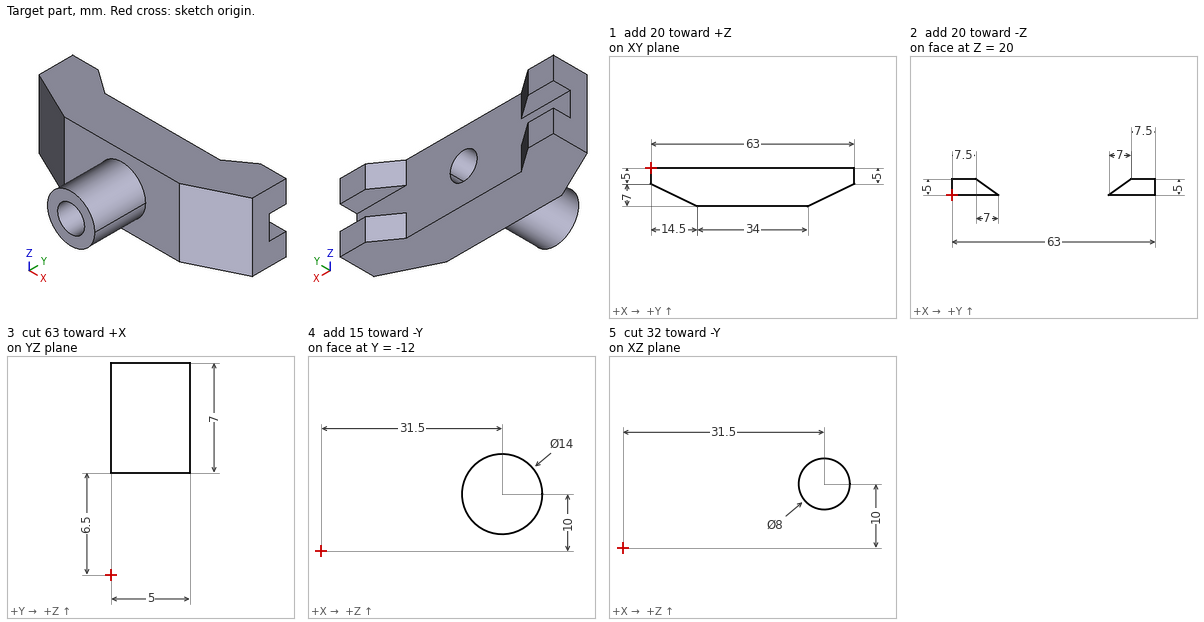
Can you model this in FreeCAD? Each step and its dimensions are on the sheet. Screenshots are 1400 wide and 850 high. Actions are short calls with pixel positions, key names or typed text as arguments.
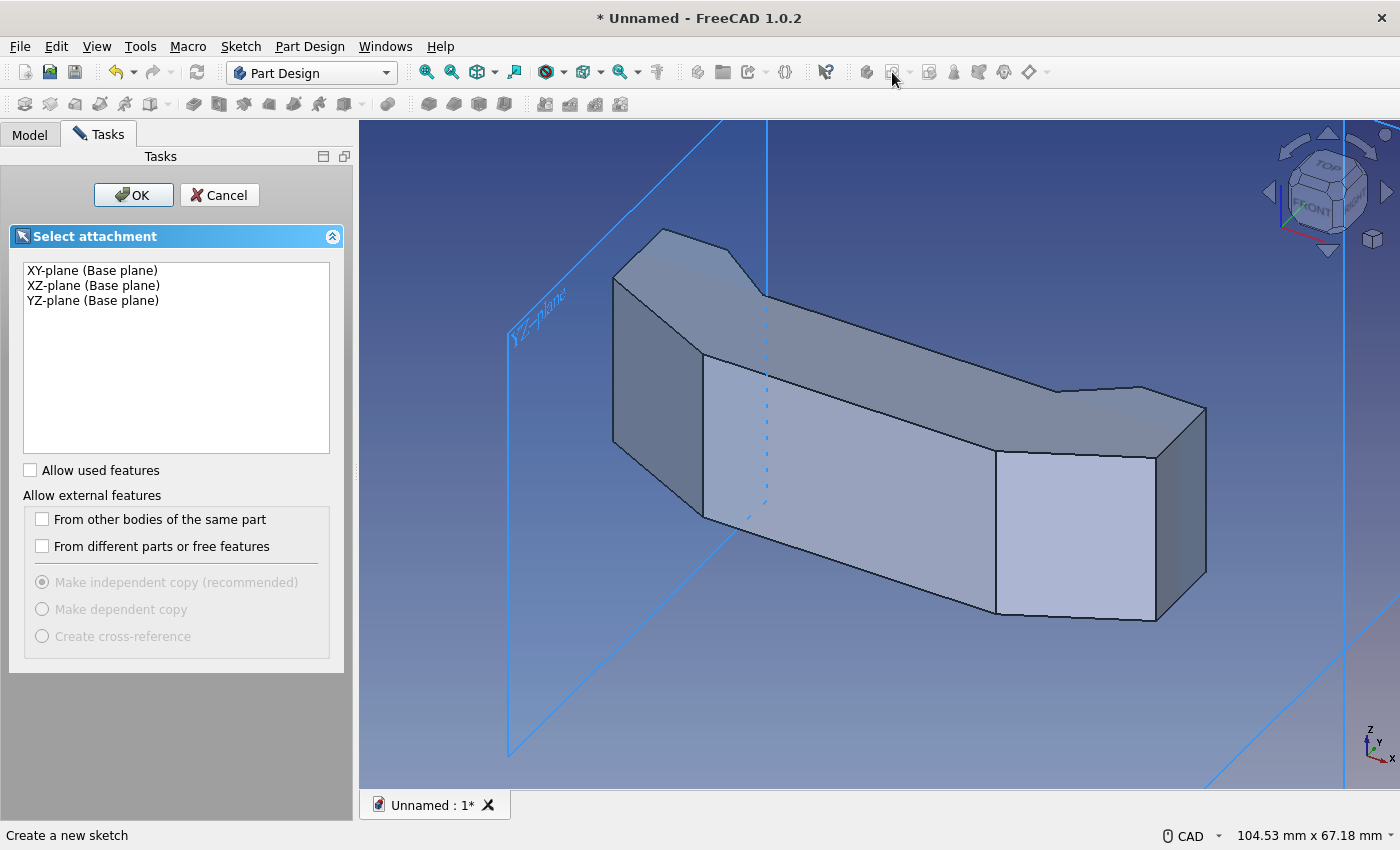
click(84, 300)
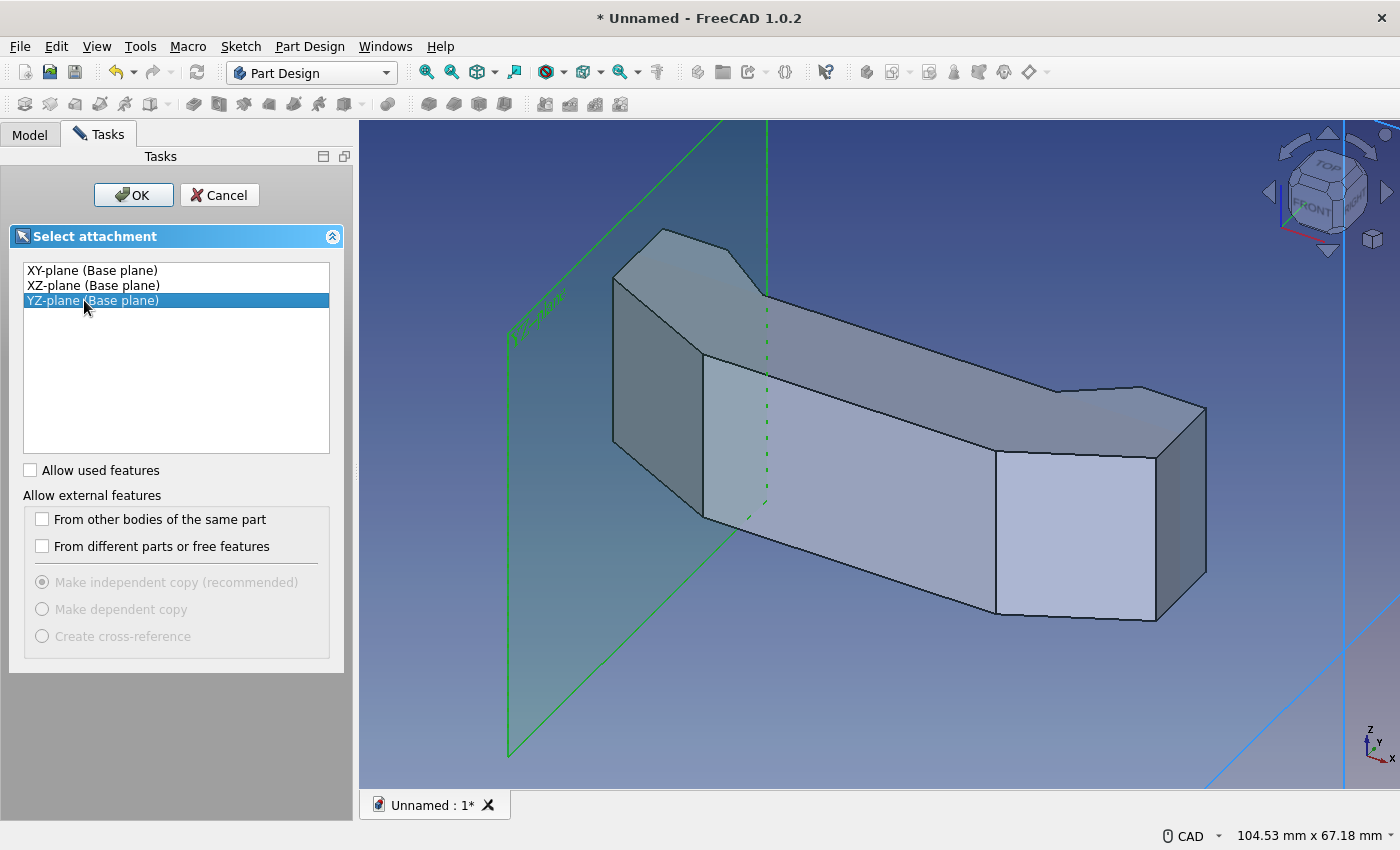
click(134, 195)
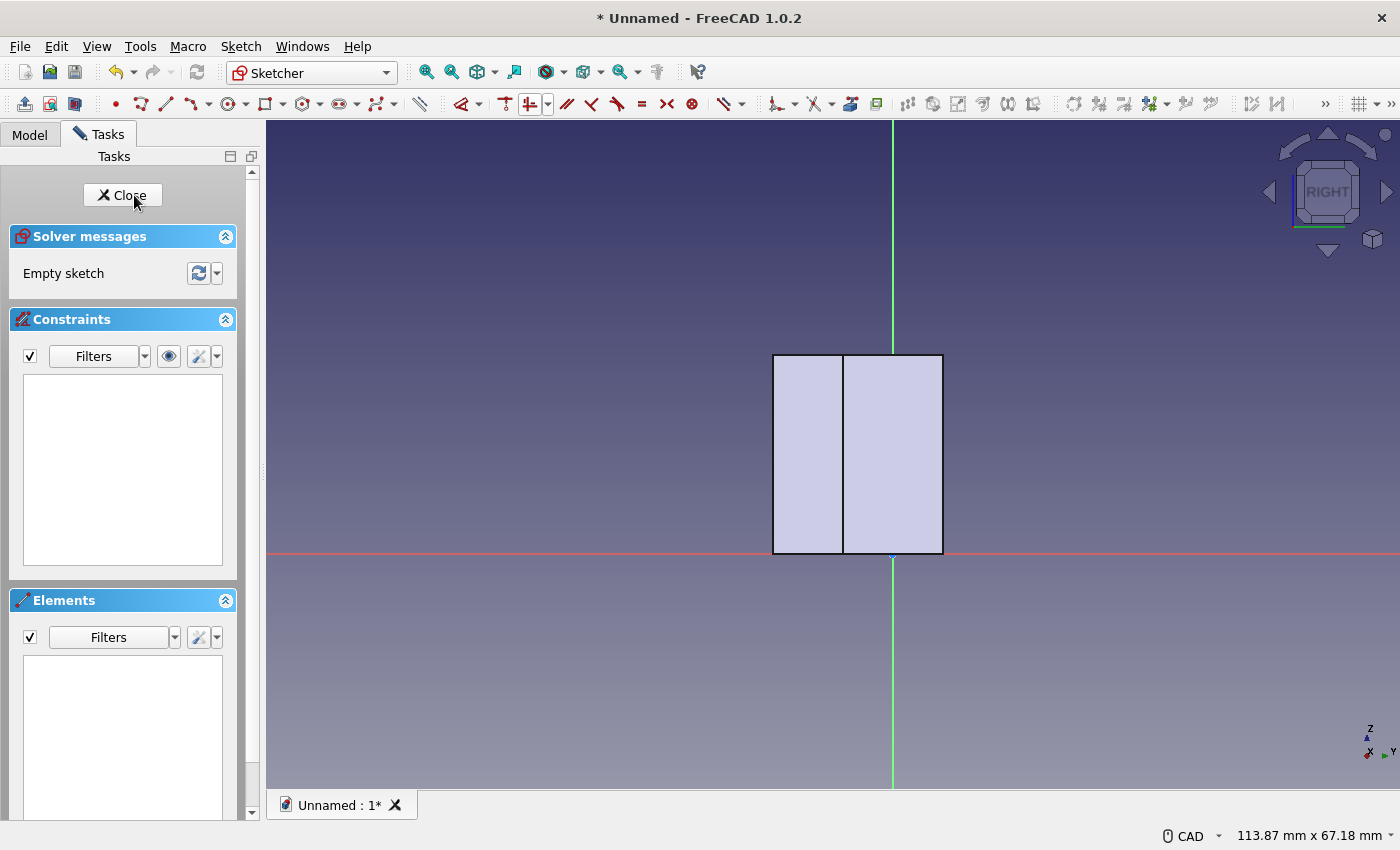
click(75, 104)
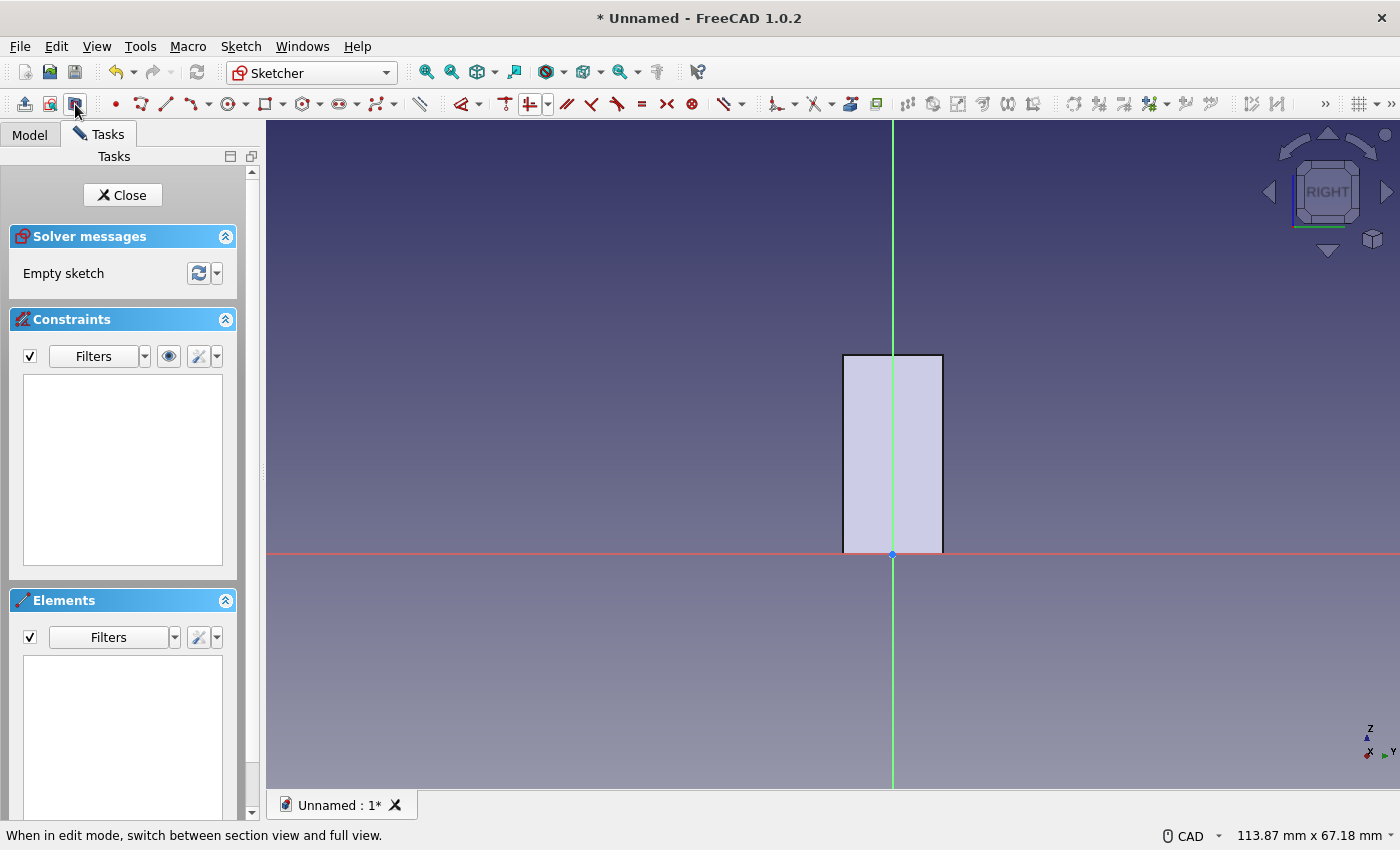
scroll(984, 501, up, 6)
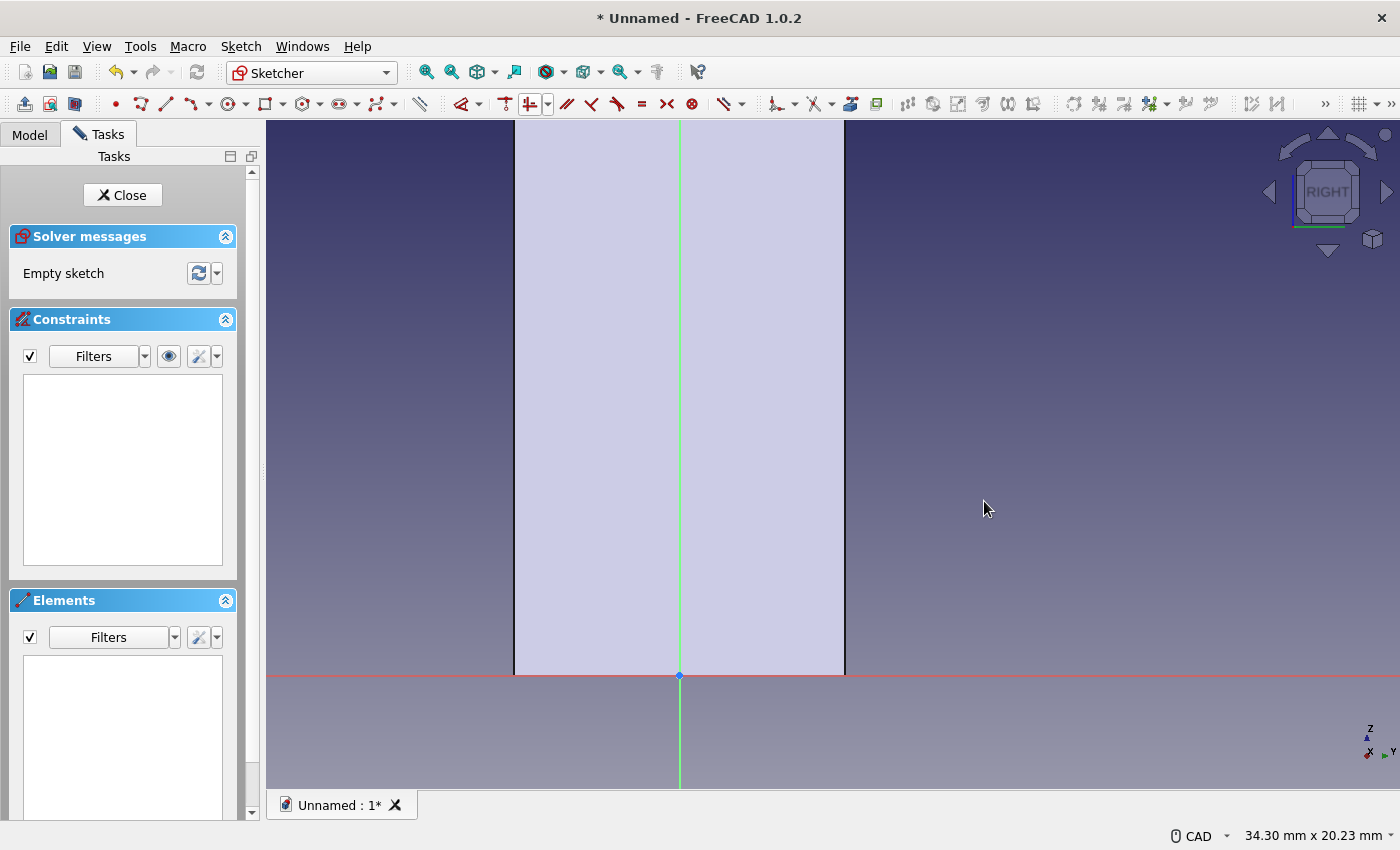
click(264, 104)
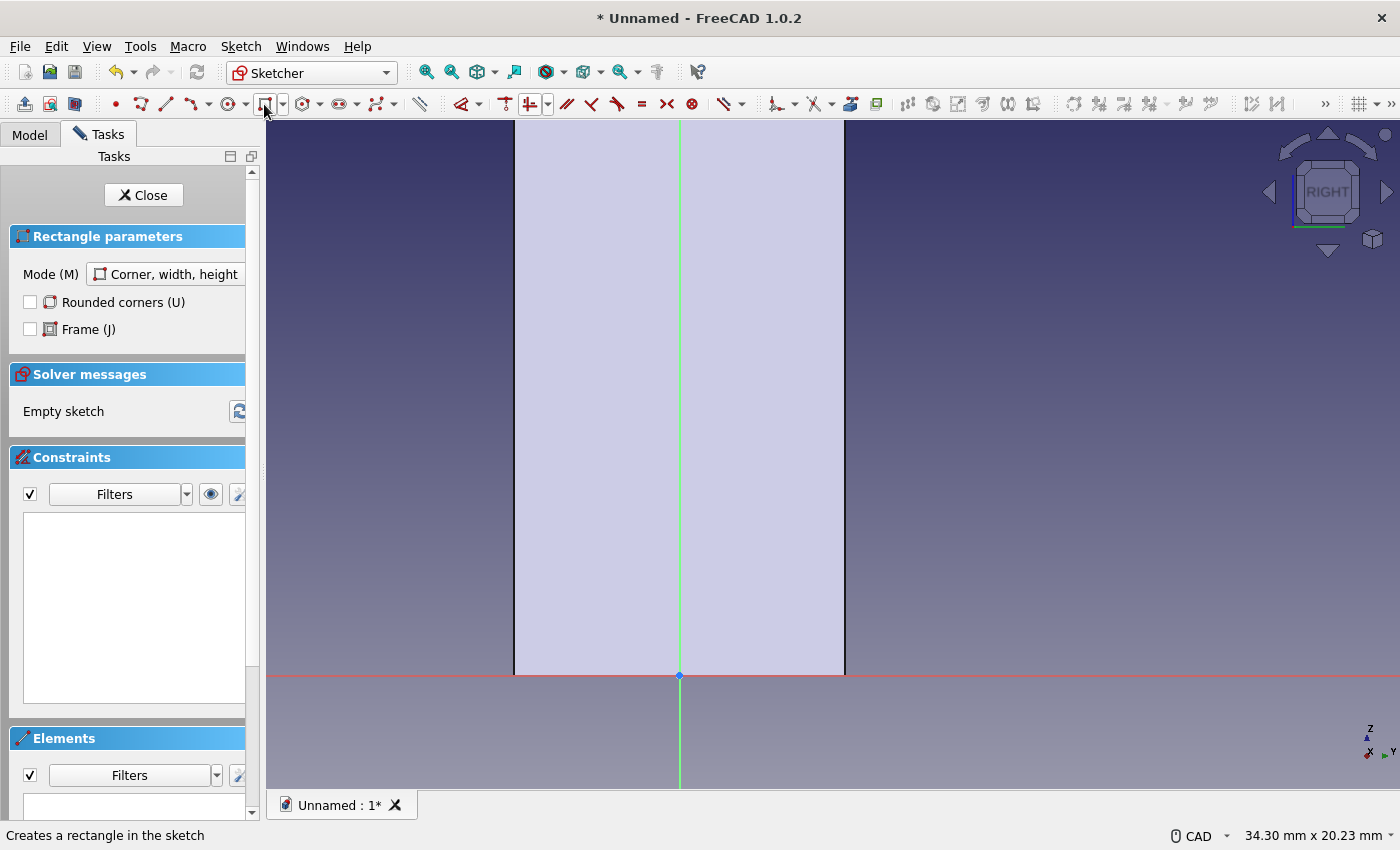
click(680, 230)
move(845, 461)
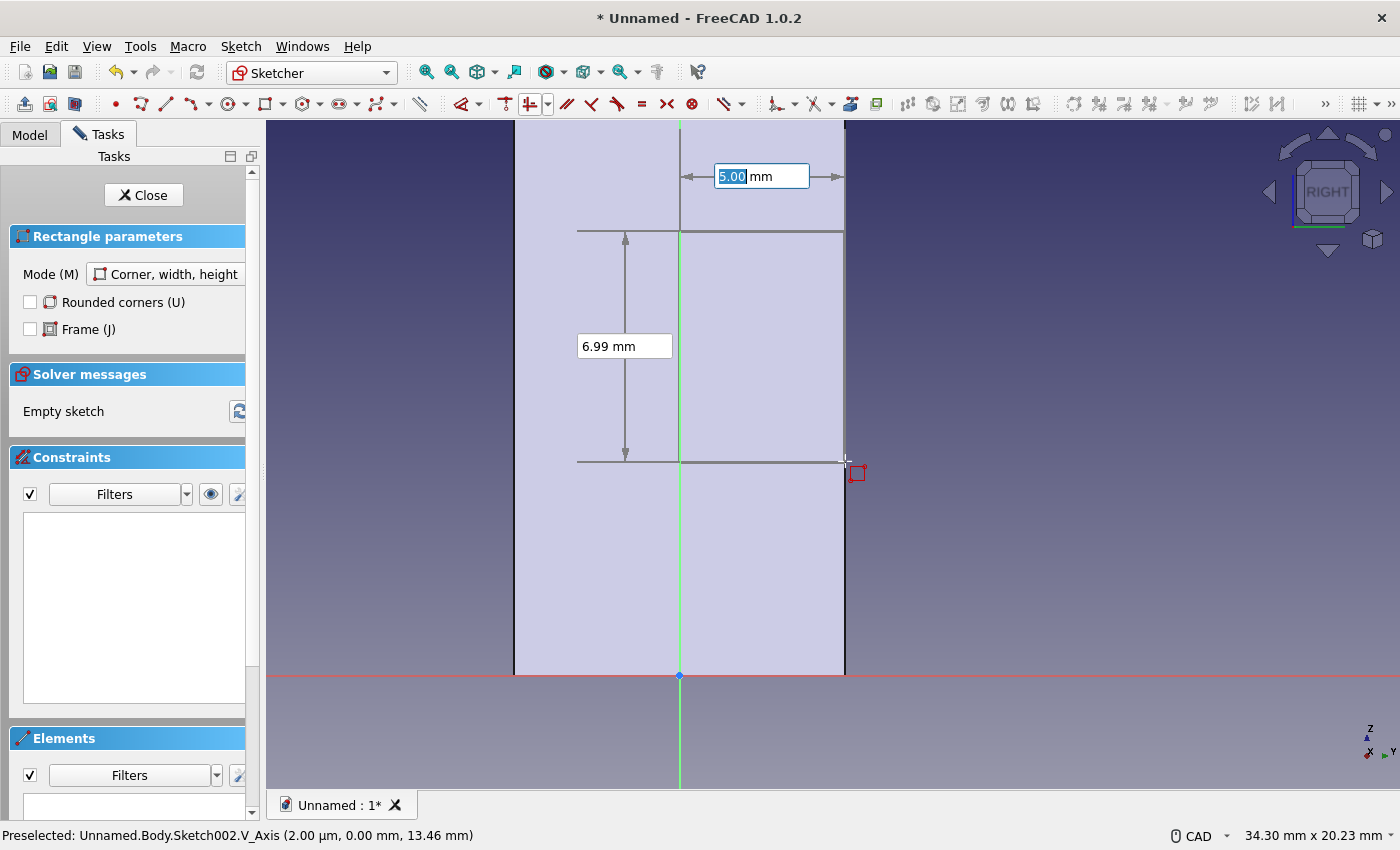
text(5)
key(Tab)
text(7)
key(Return)
key(Escape)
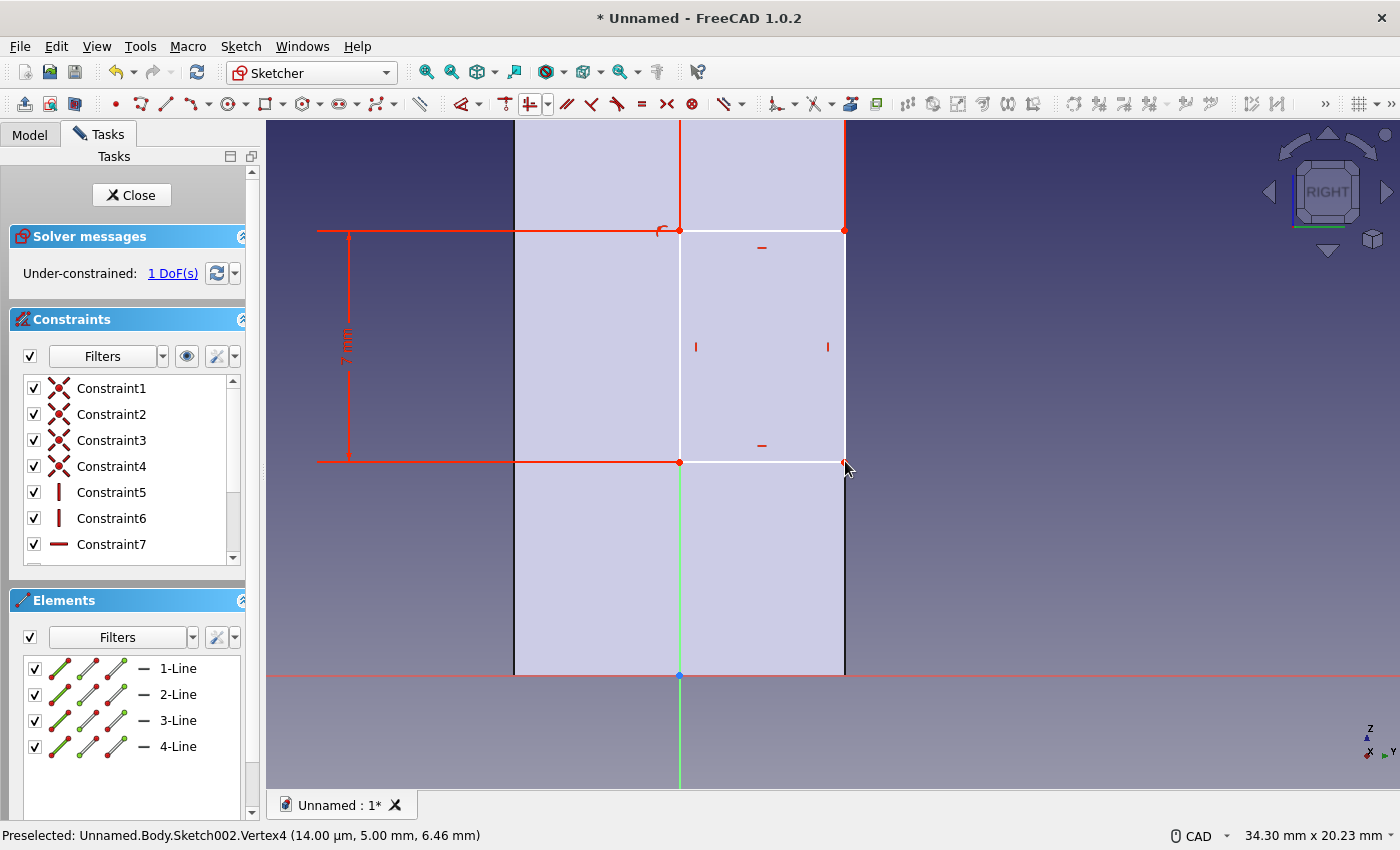
click(460, 104)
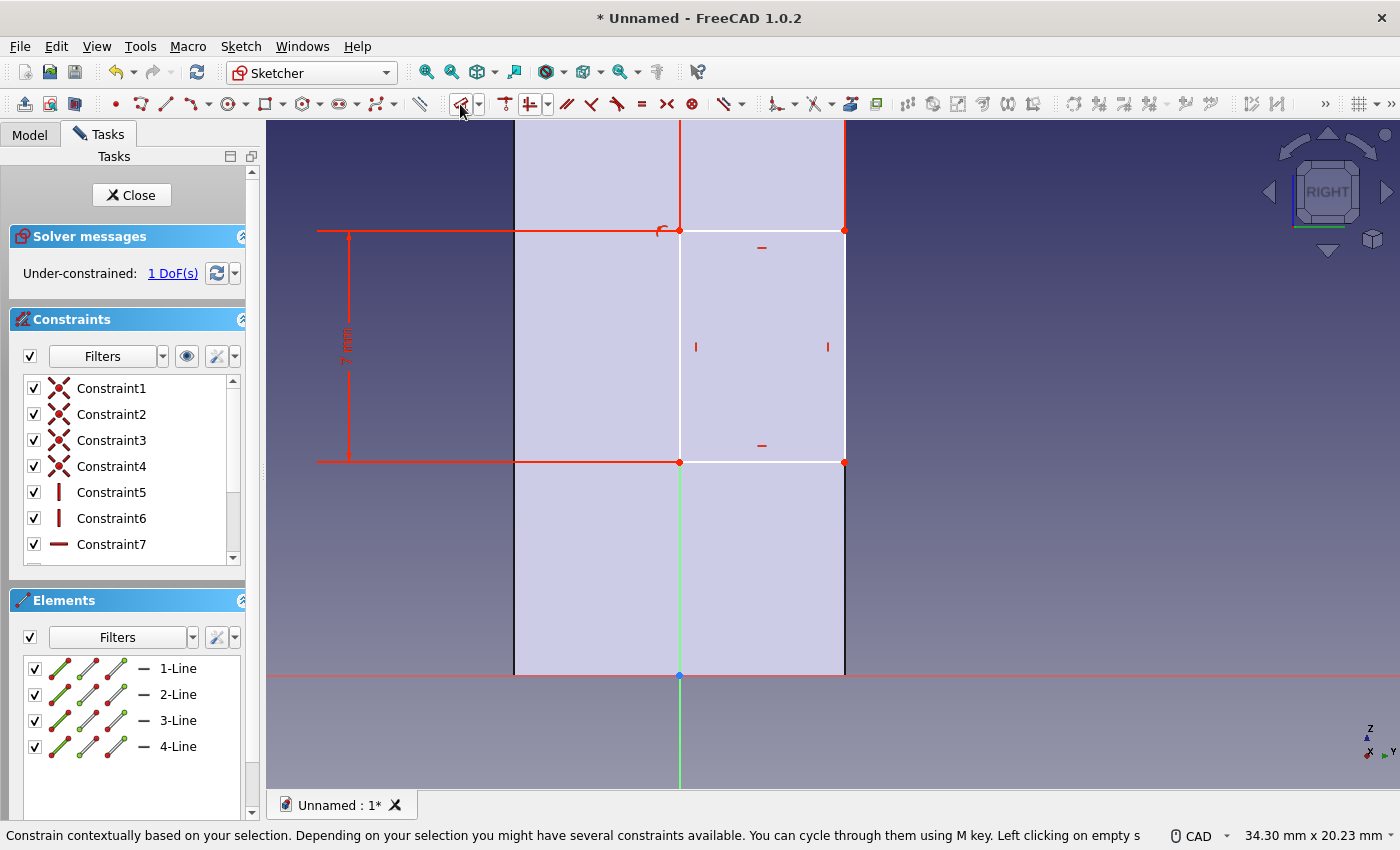
click(680, 462)
click(646, 569)